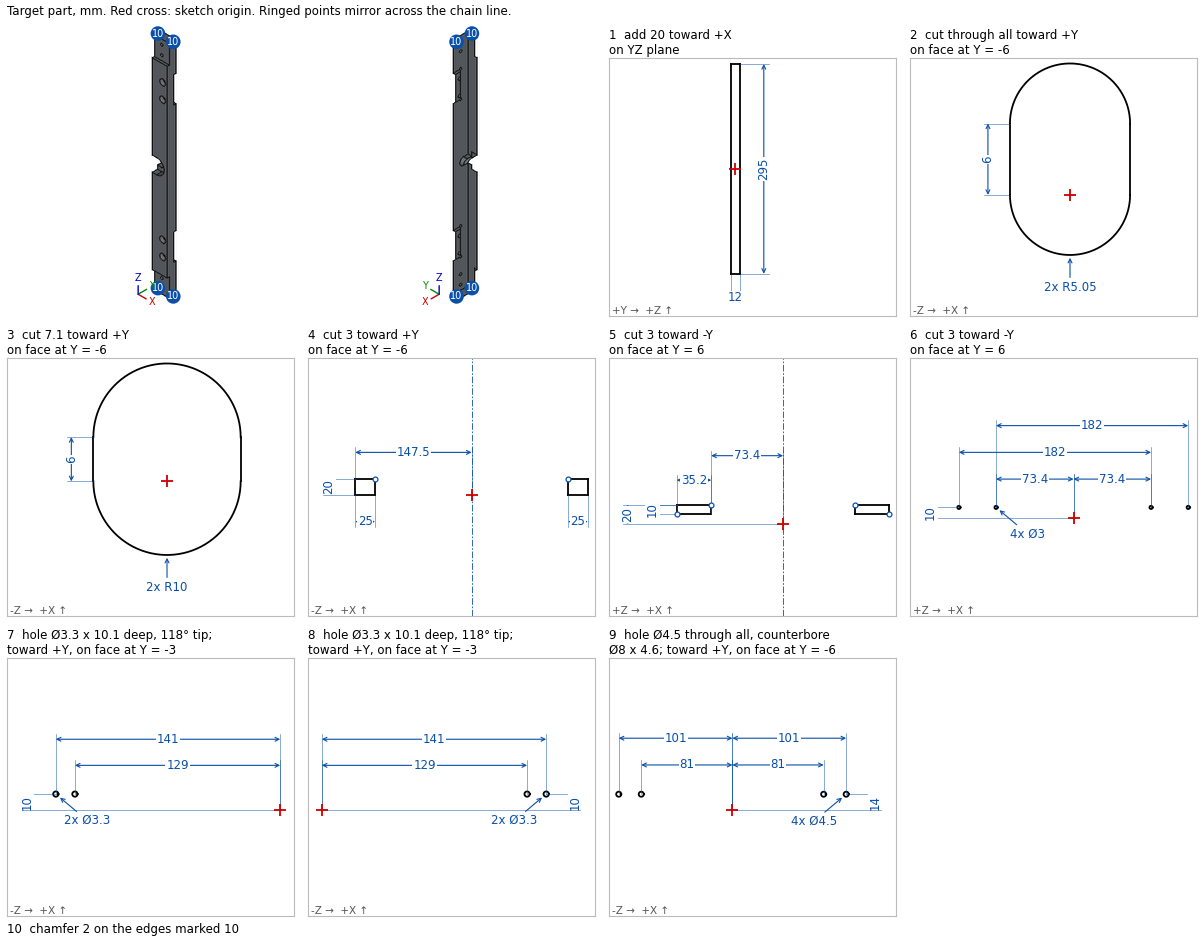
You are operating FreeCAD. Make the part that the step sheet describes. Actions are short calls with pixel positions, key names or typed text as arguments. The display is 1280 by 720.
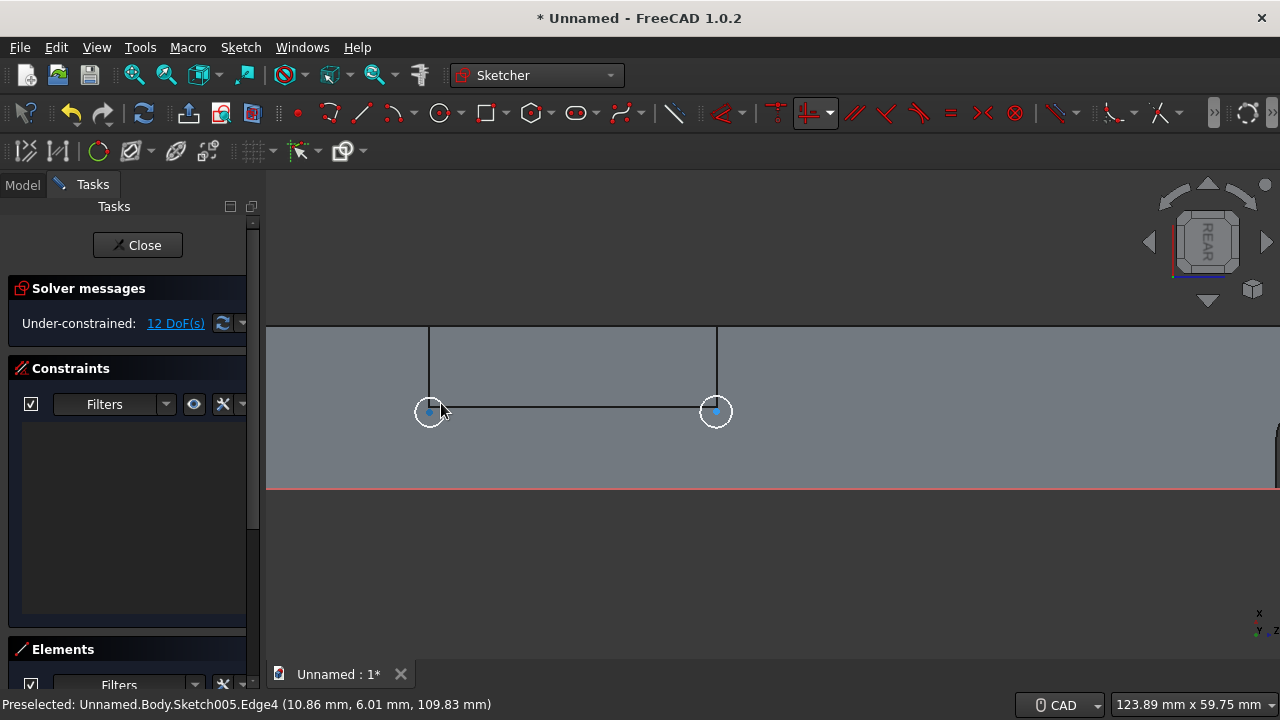
click(440, 402)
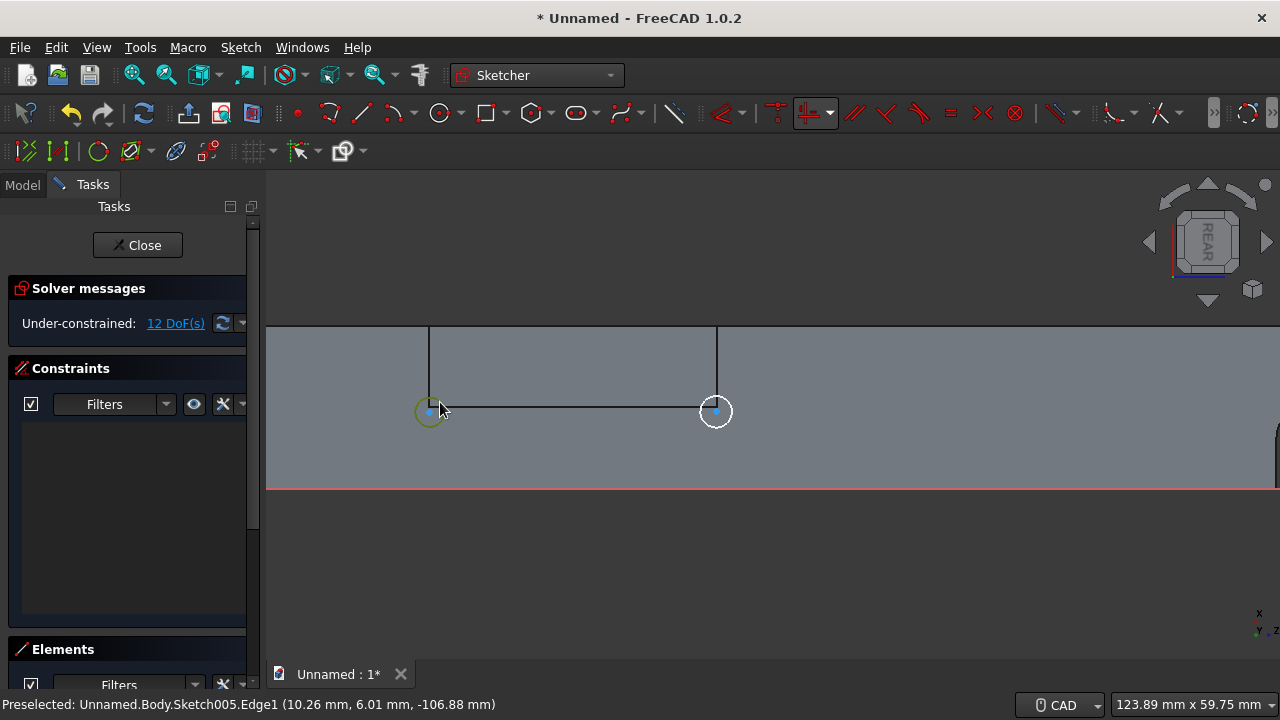
click(727, 401)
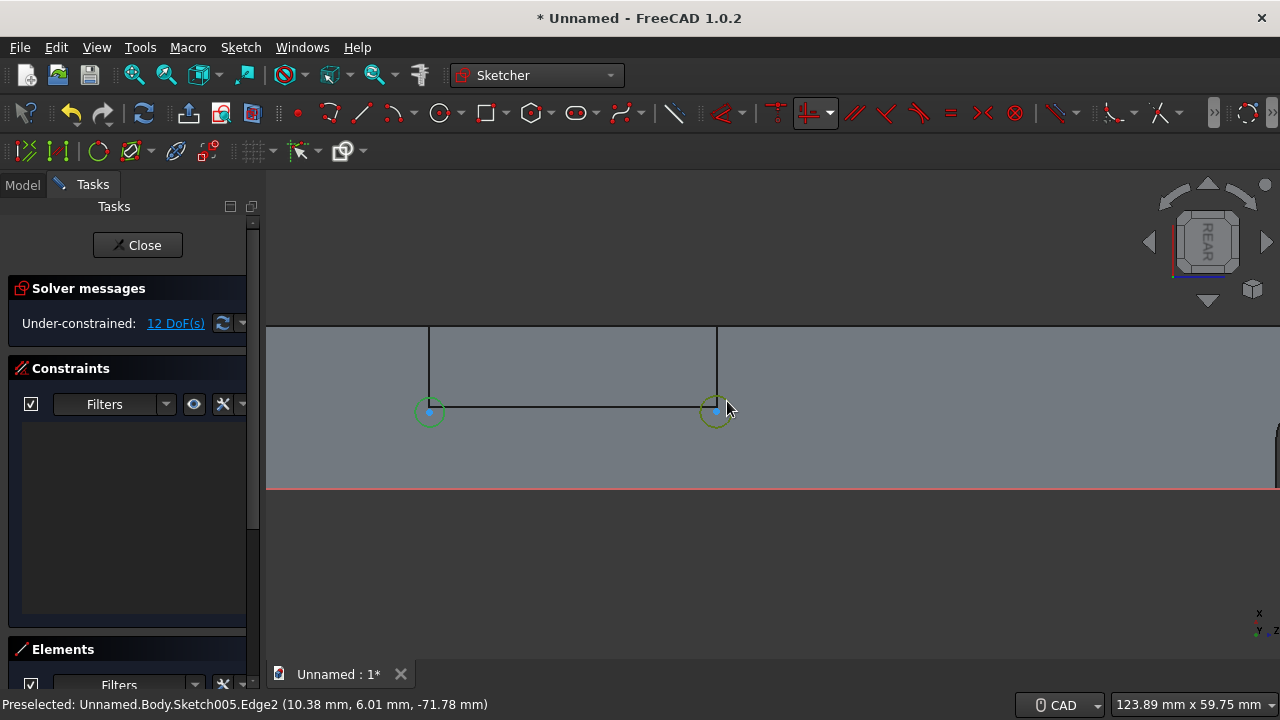
scroll(440, 403, down, 6)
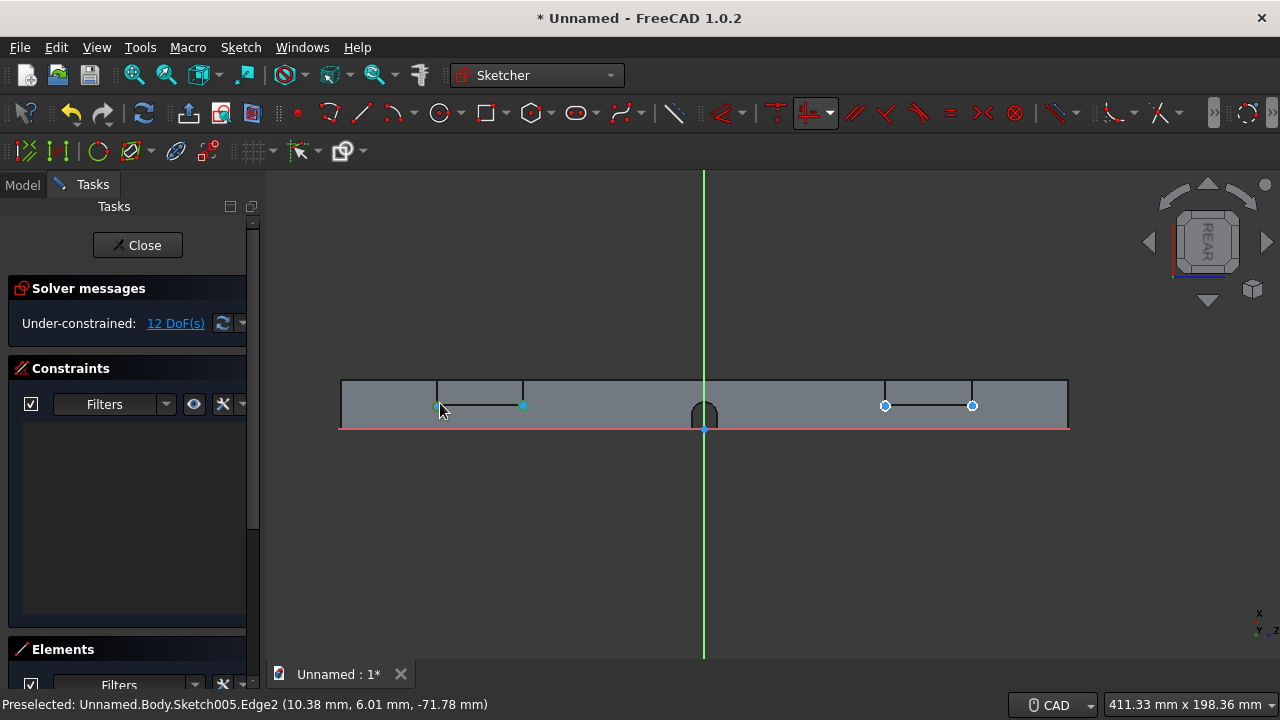
scroll(889, 403, up, 6)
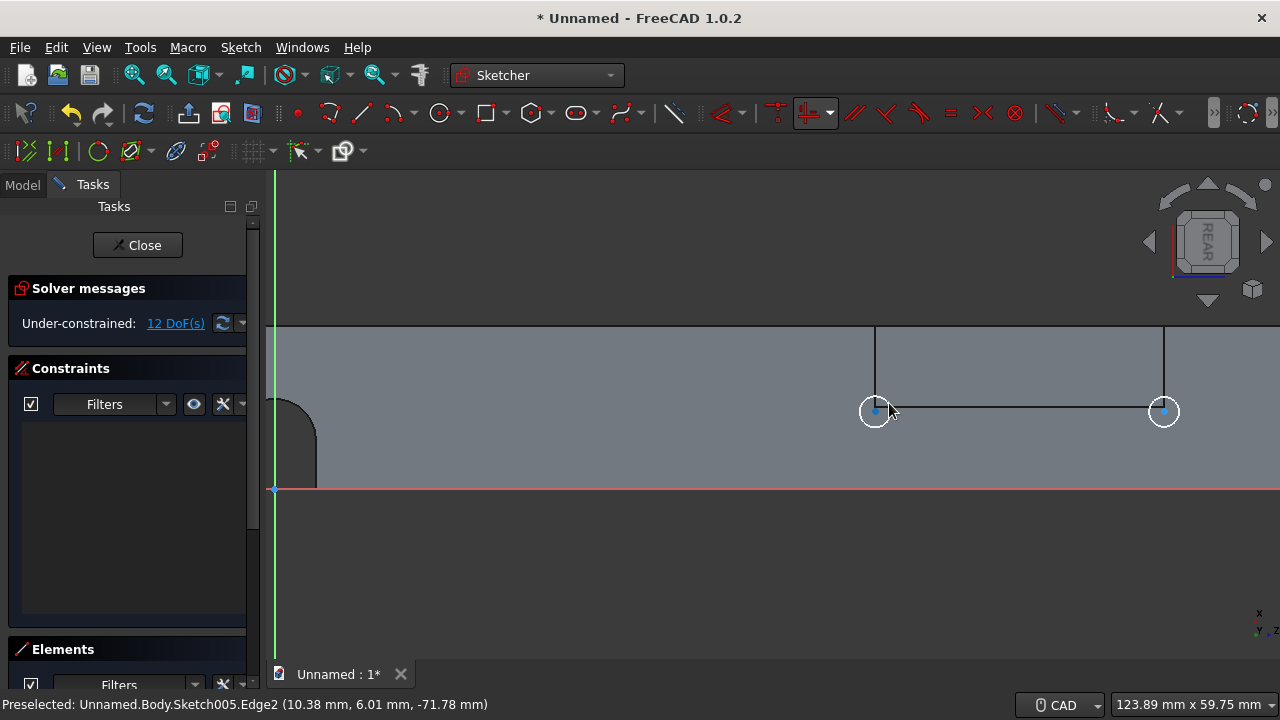
click(886, 401)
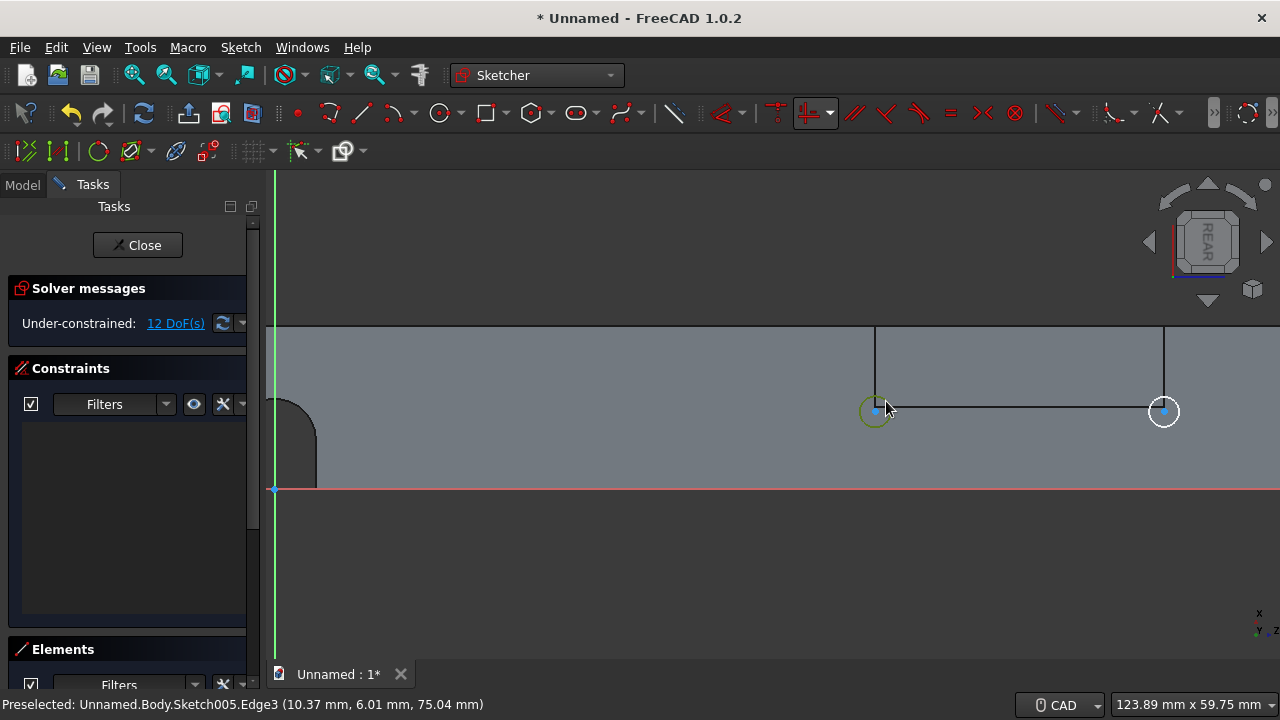
scroll(890, 403, down, 6)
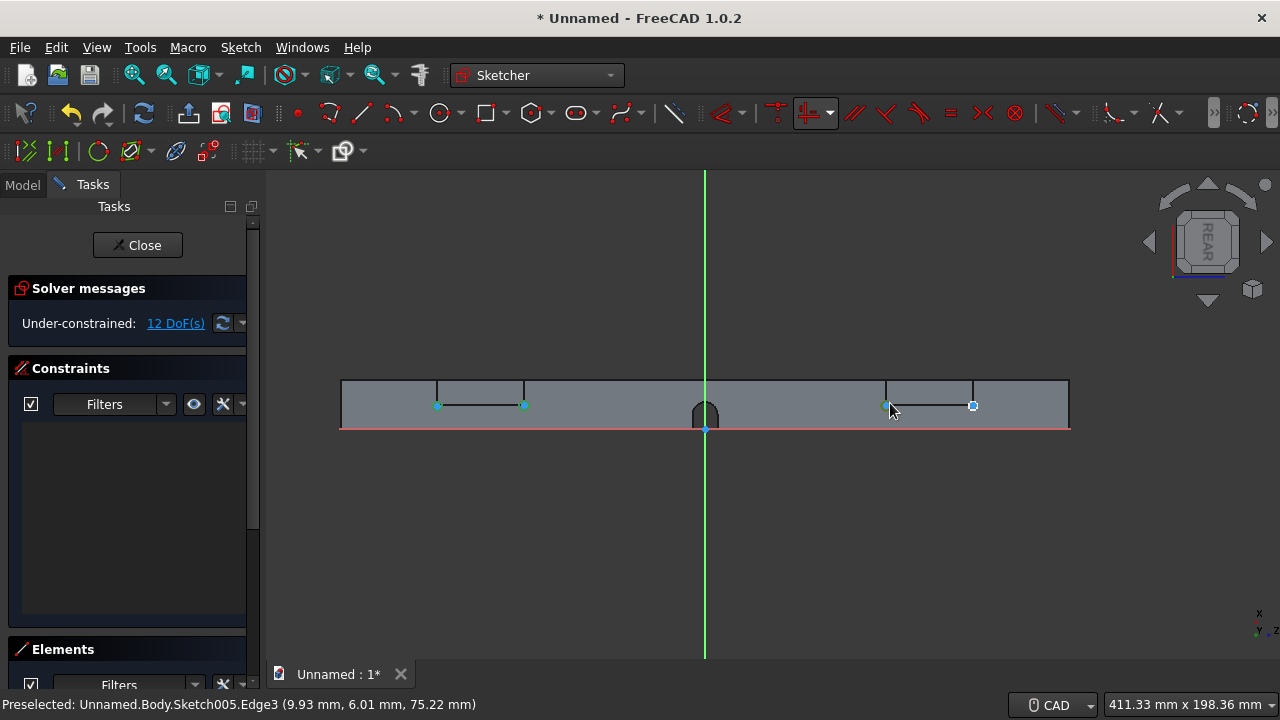
scroll(976, 403, up, 6)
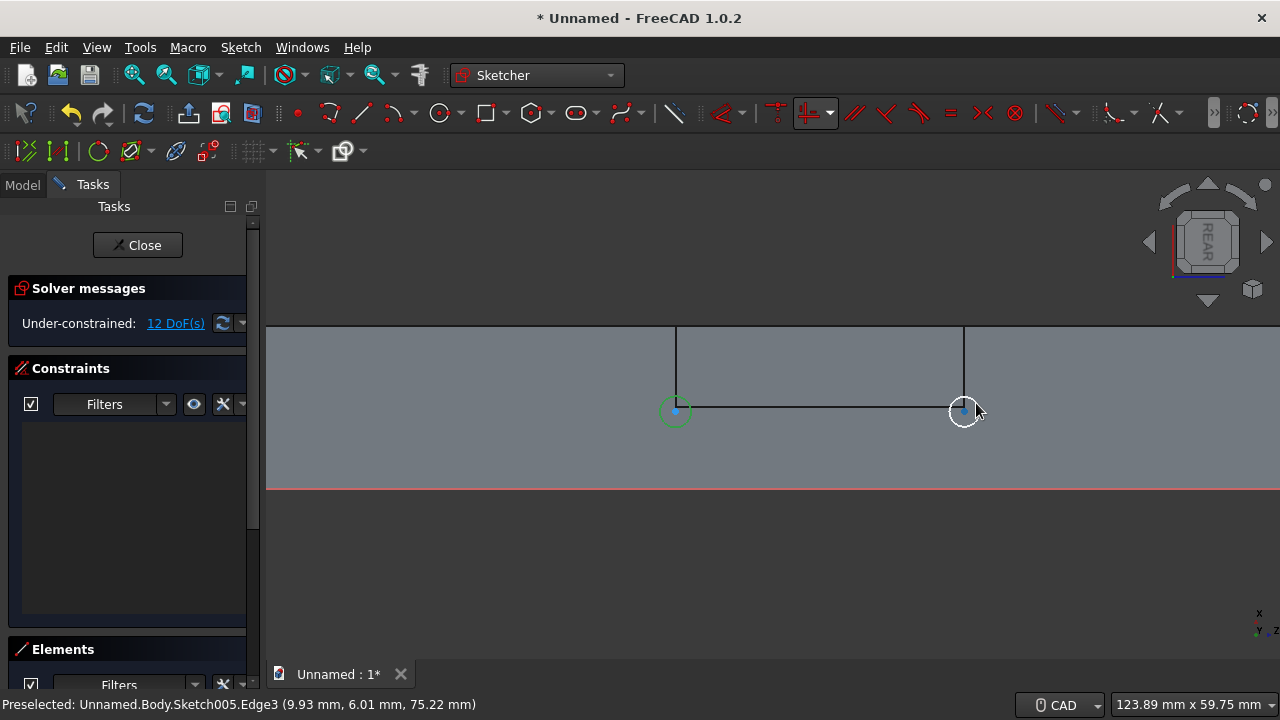
click(975, 401)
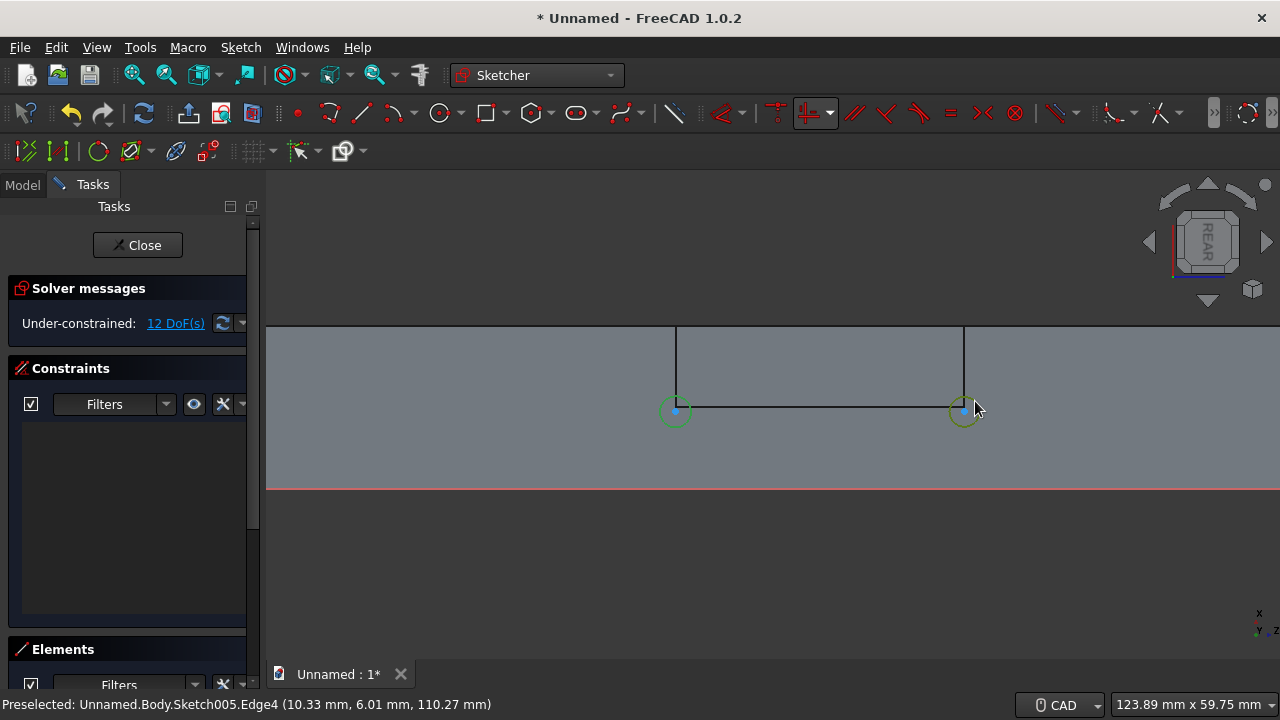
click(952, 114)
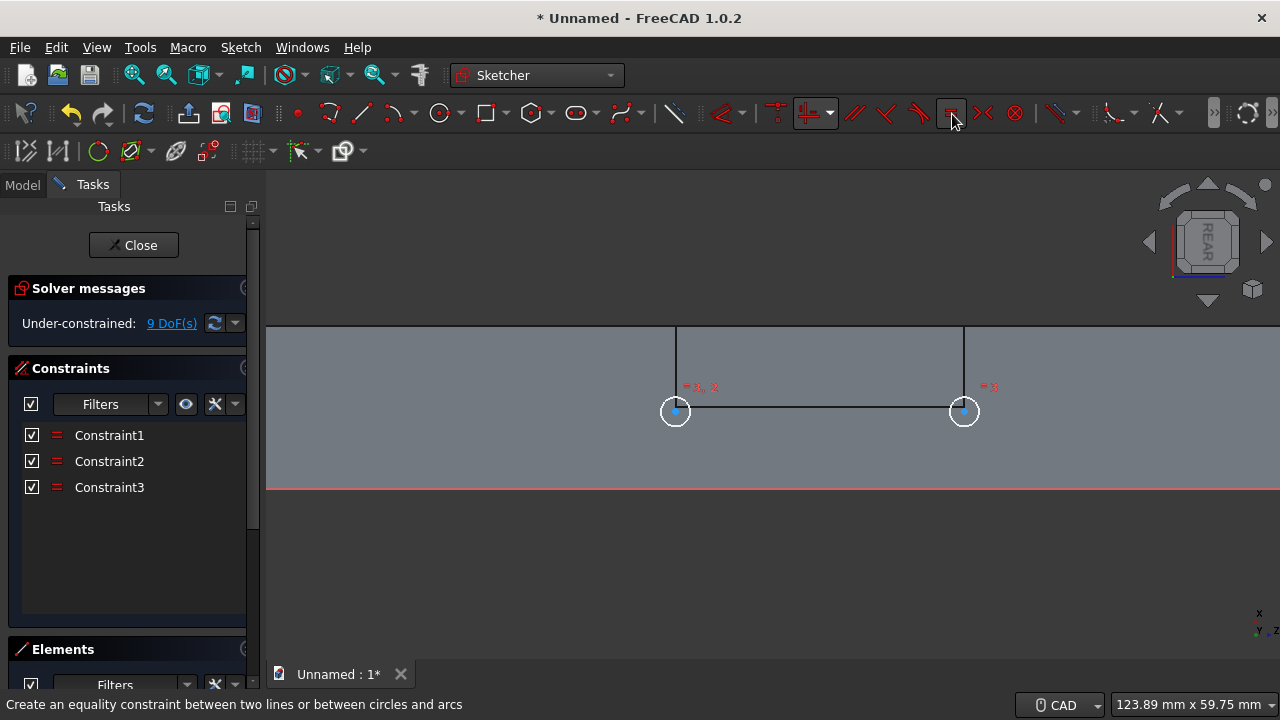
scroll(976, 403, down, 6)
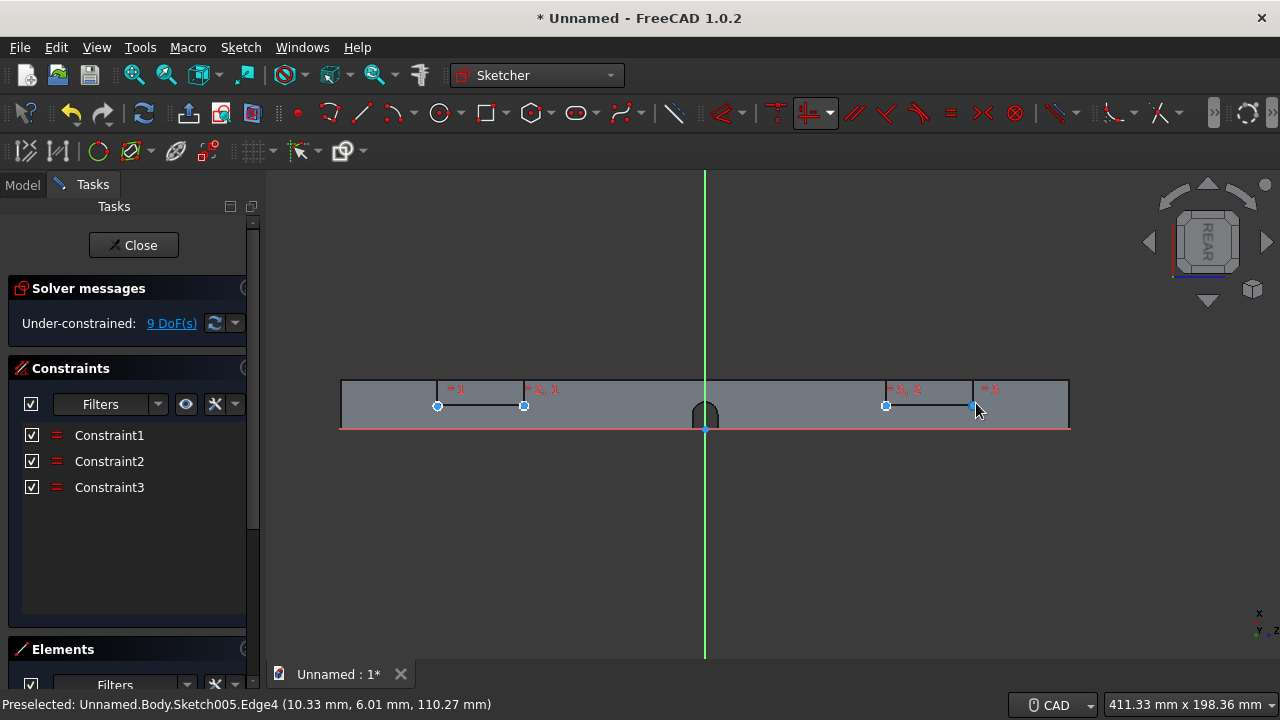
click(438, 406)